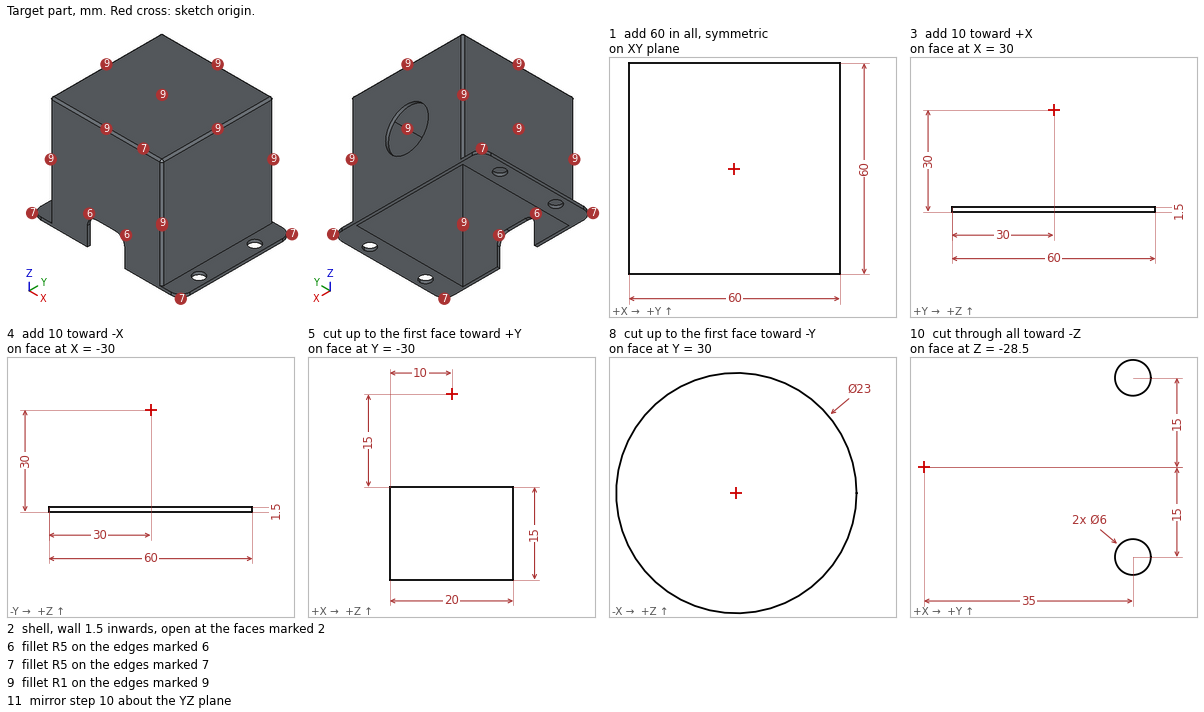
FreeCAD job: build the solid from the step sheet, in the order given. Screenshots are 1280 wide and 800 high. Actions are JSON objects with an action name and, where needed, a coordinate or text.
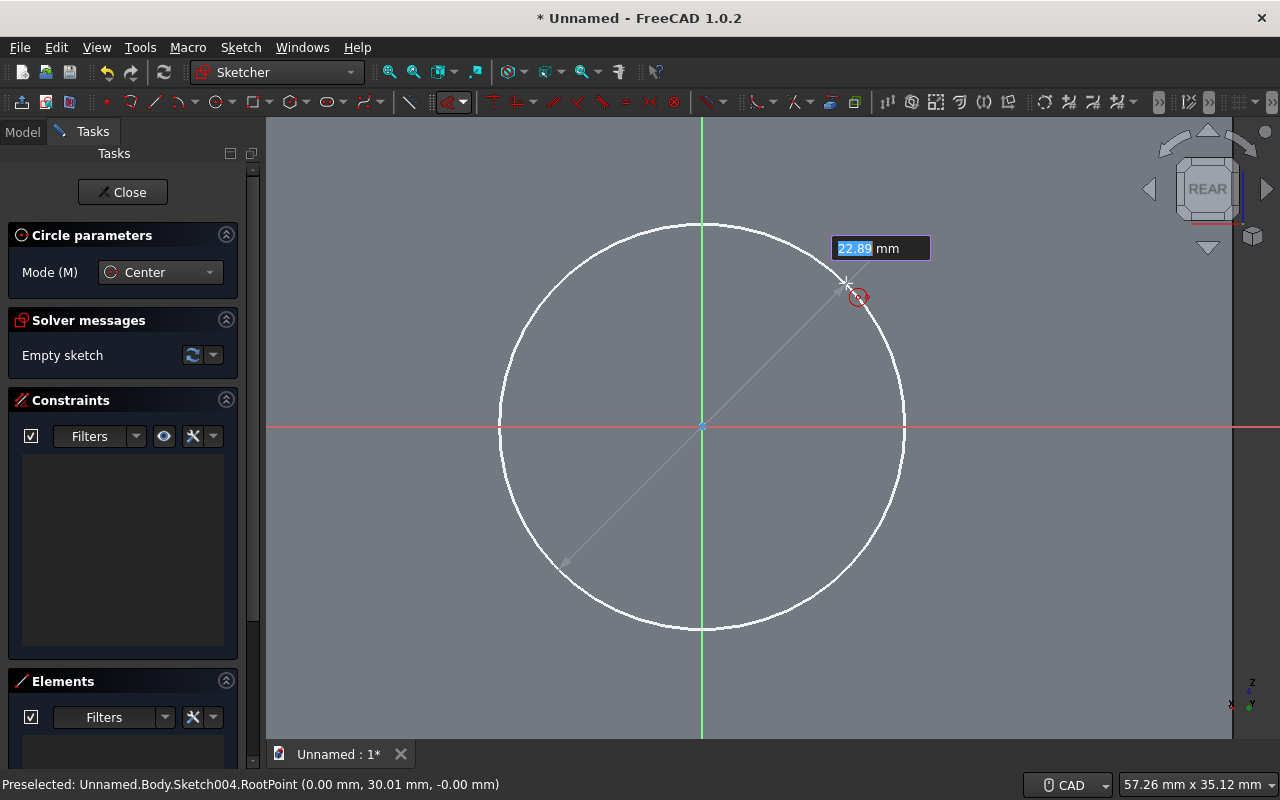
{"action": "type", "text": "23"}
{"action": "key", "text": "Return"}
{"action": "key", "text": "Escape"}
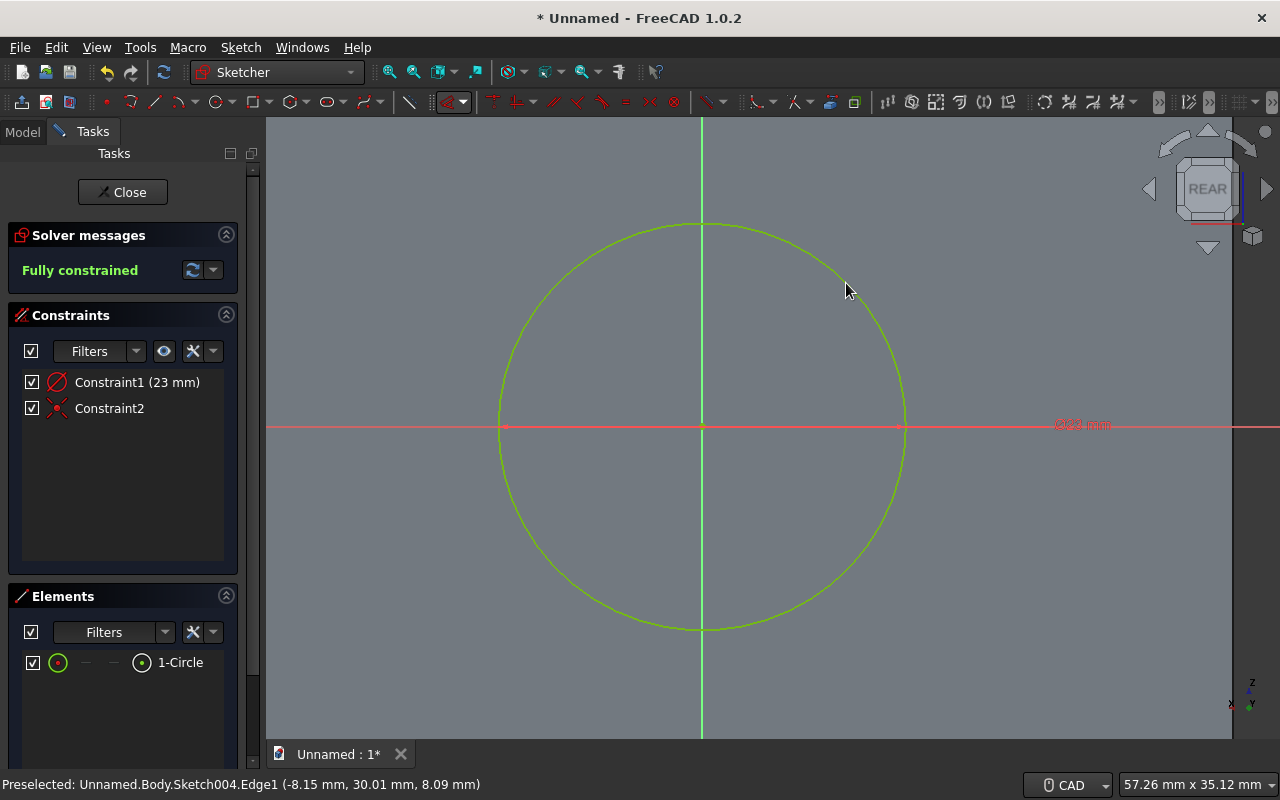
{"action": "left_click", "coordinate": [123, 192]}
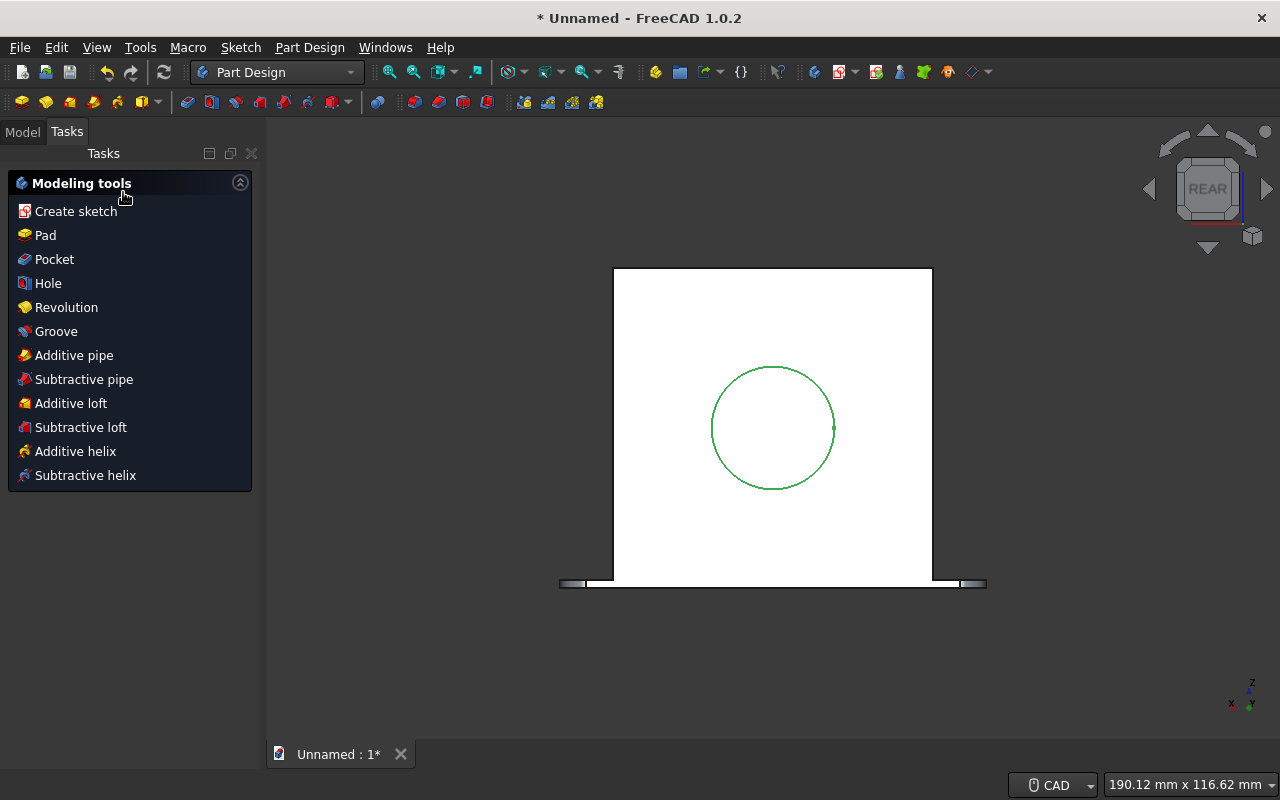
{"action": "left_click", "coordinate": [188, 102]}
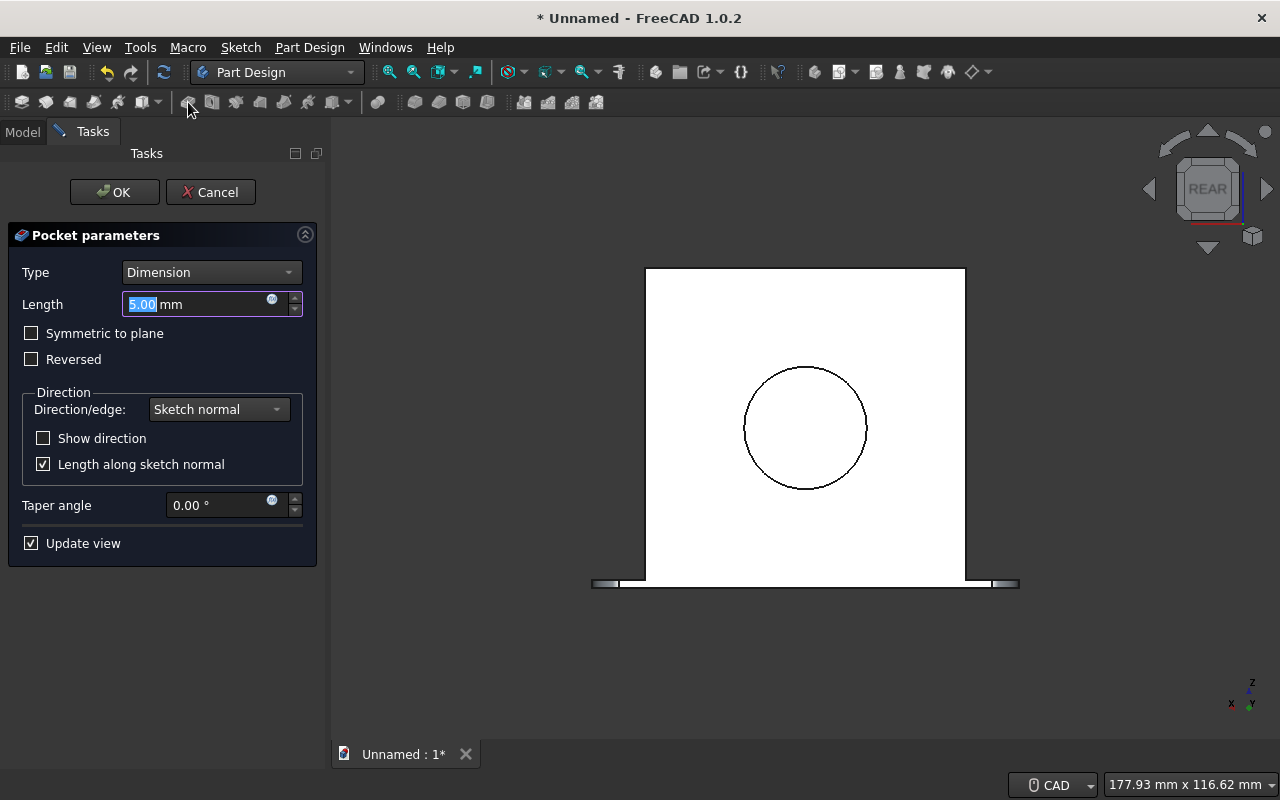
{"action": "left_click", "coordinate": [212, 272]}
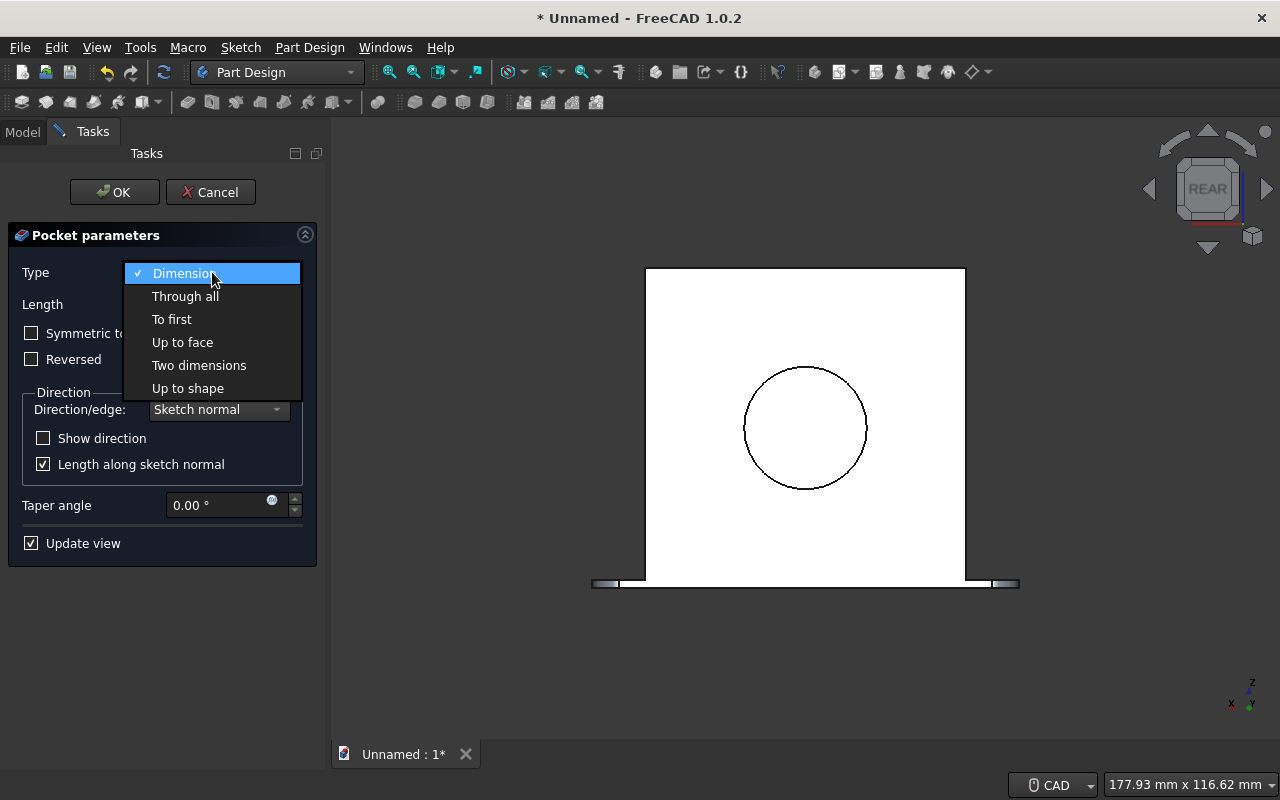
{"action": "left_click", "coordinate": [212, 320]}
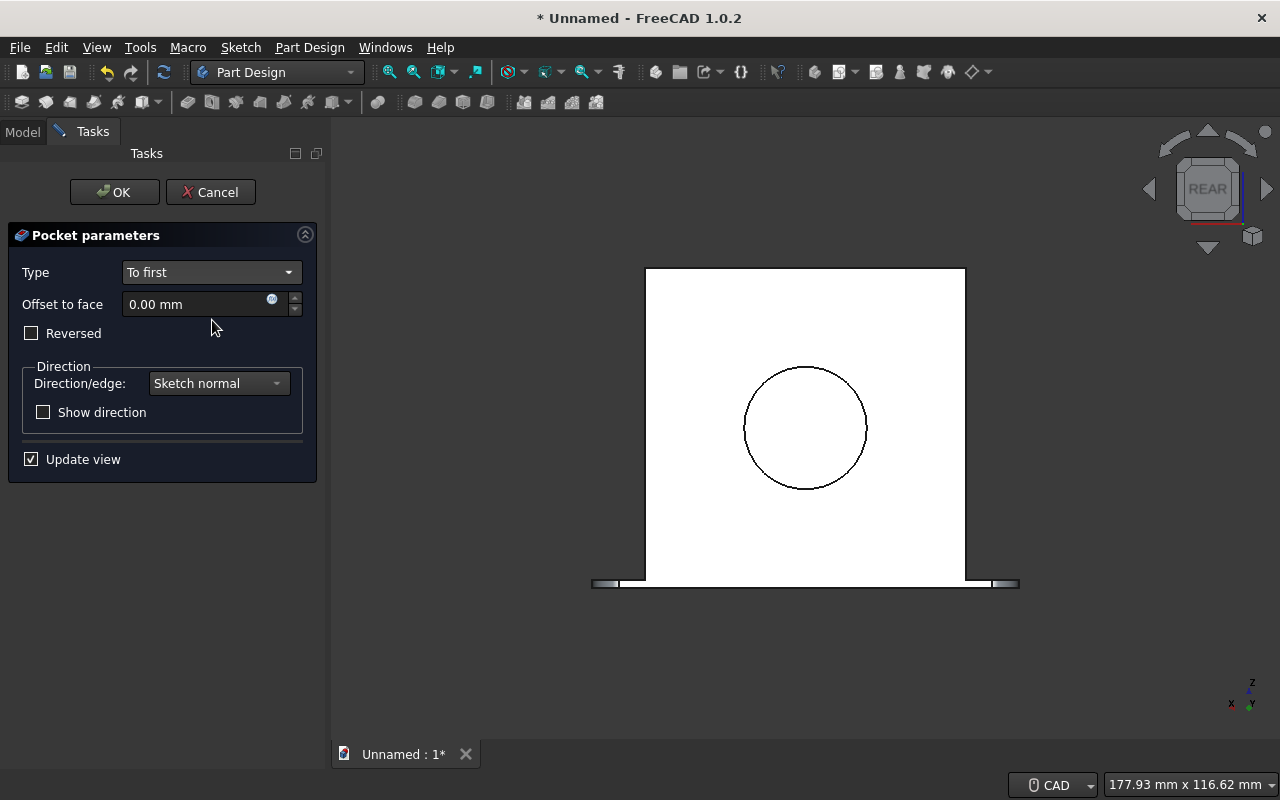
{"action": "left_click", "coordinate": [115, 192]}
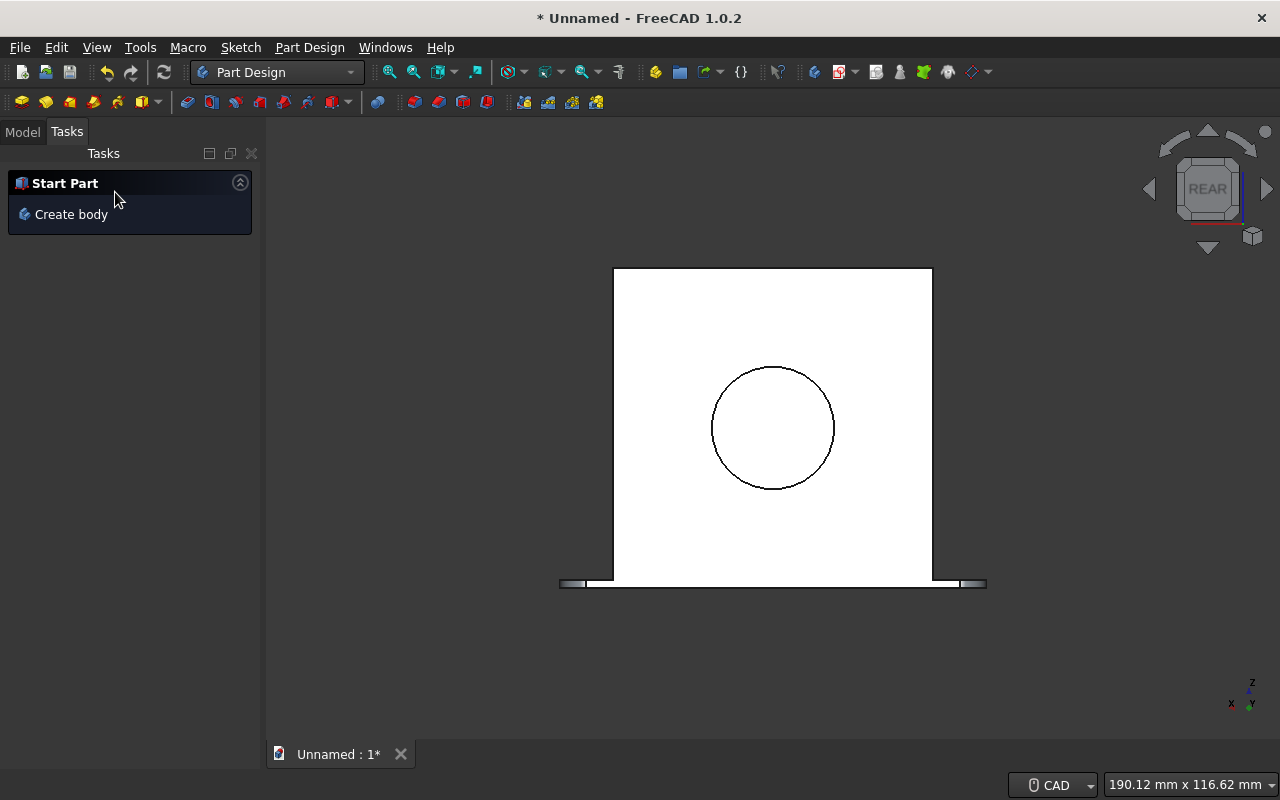
{"action": "left_click", "coordinate": [933, 423]}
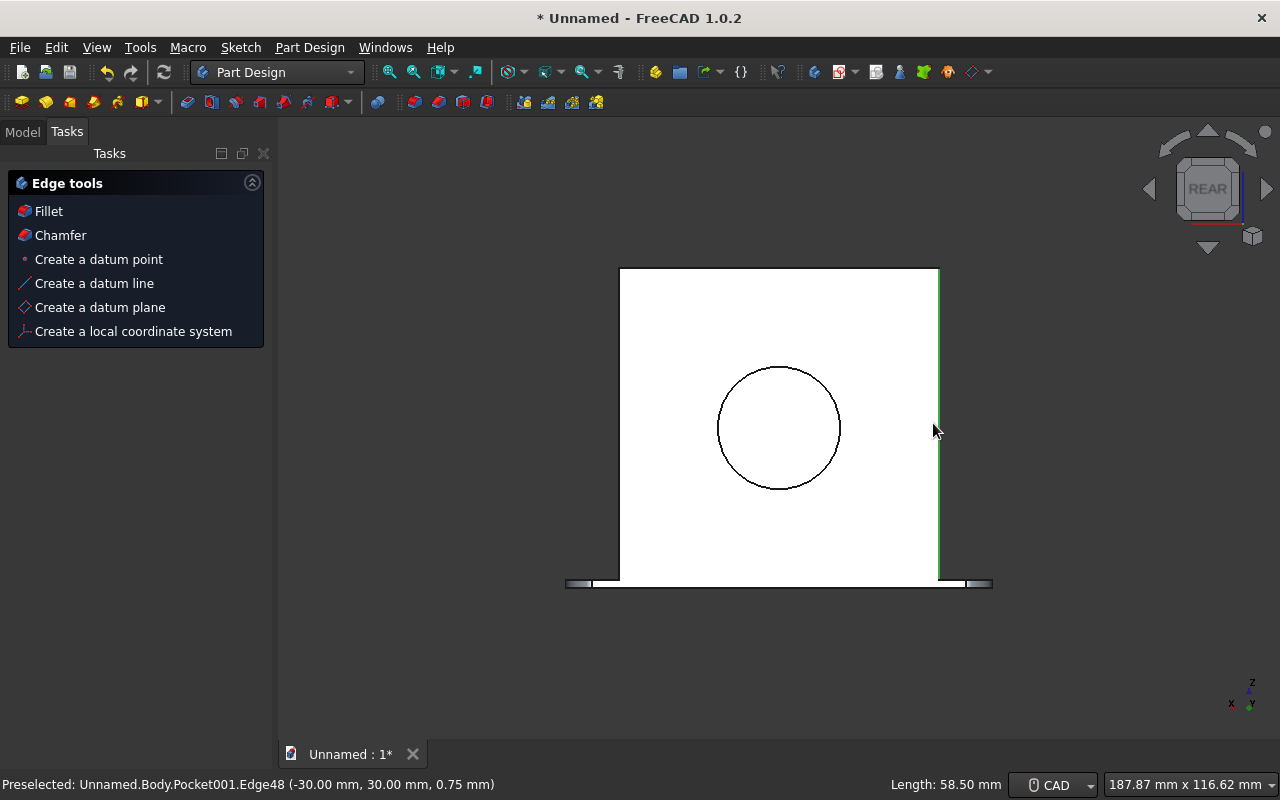
{"action": "key", "text": "0"}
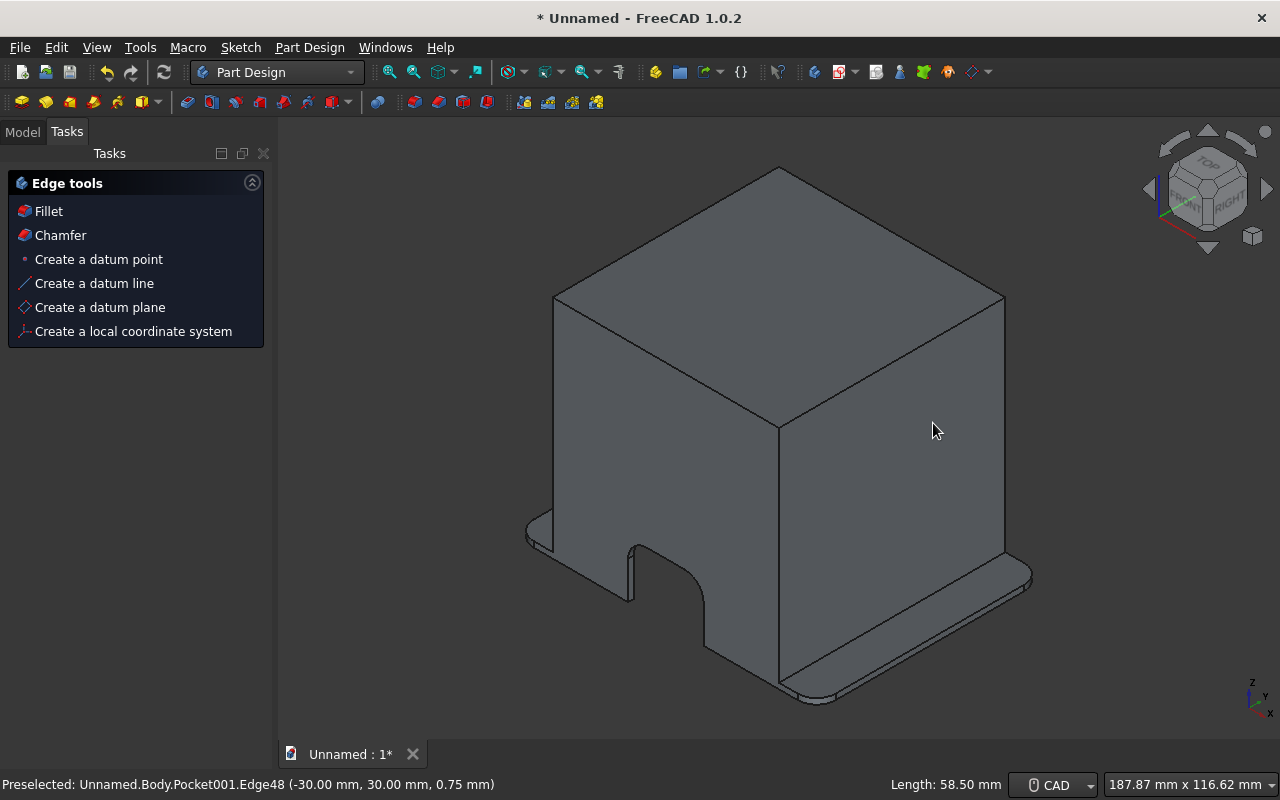
{"action": "left_click", "coordinate": [779, 296], "text": "ctrl"}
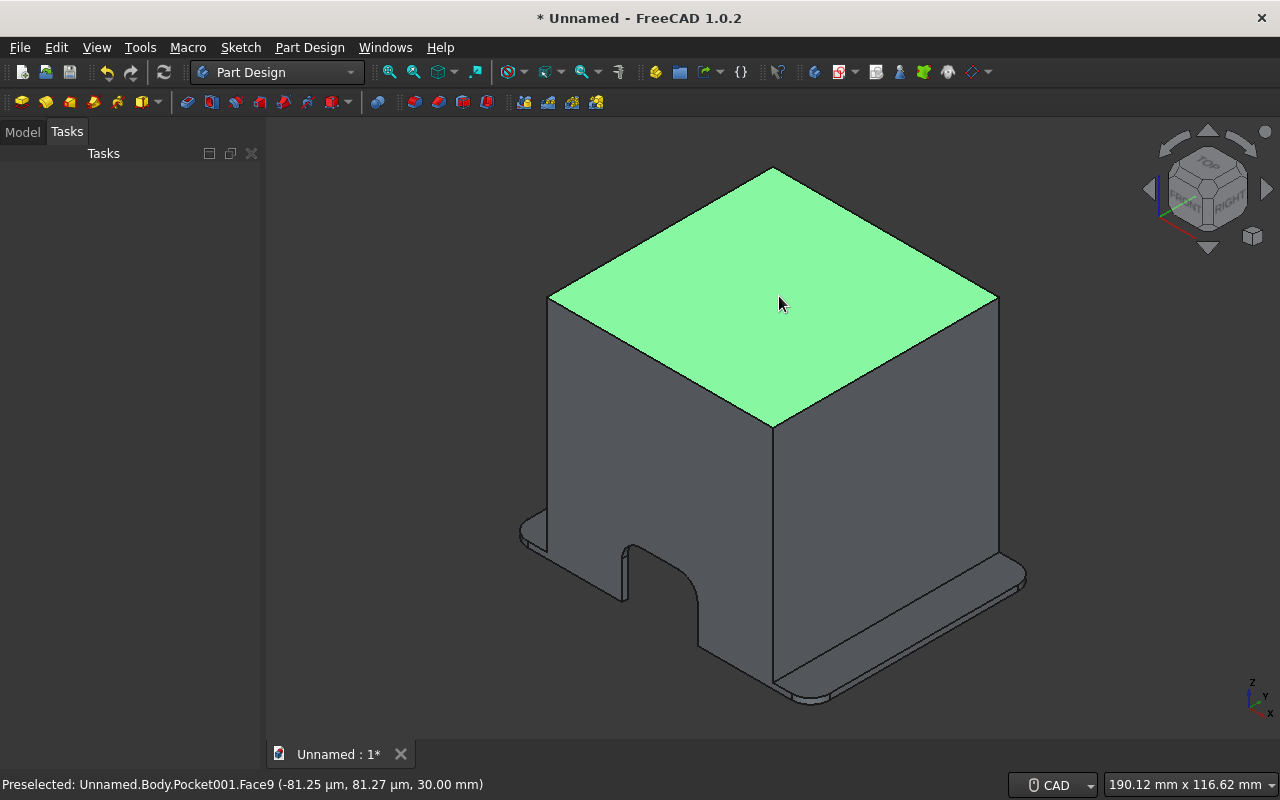
{"action": "left_click", "coordinate": [773, 554], "text": "ctrl"}